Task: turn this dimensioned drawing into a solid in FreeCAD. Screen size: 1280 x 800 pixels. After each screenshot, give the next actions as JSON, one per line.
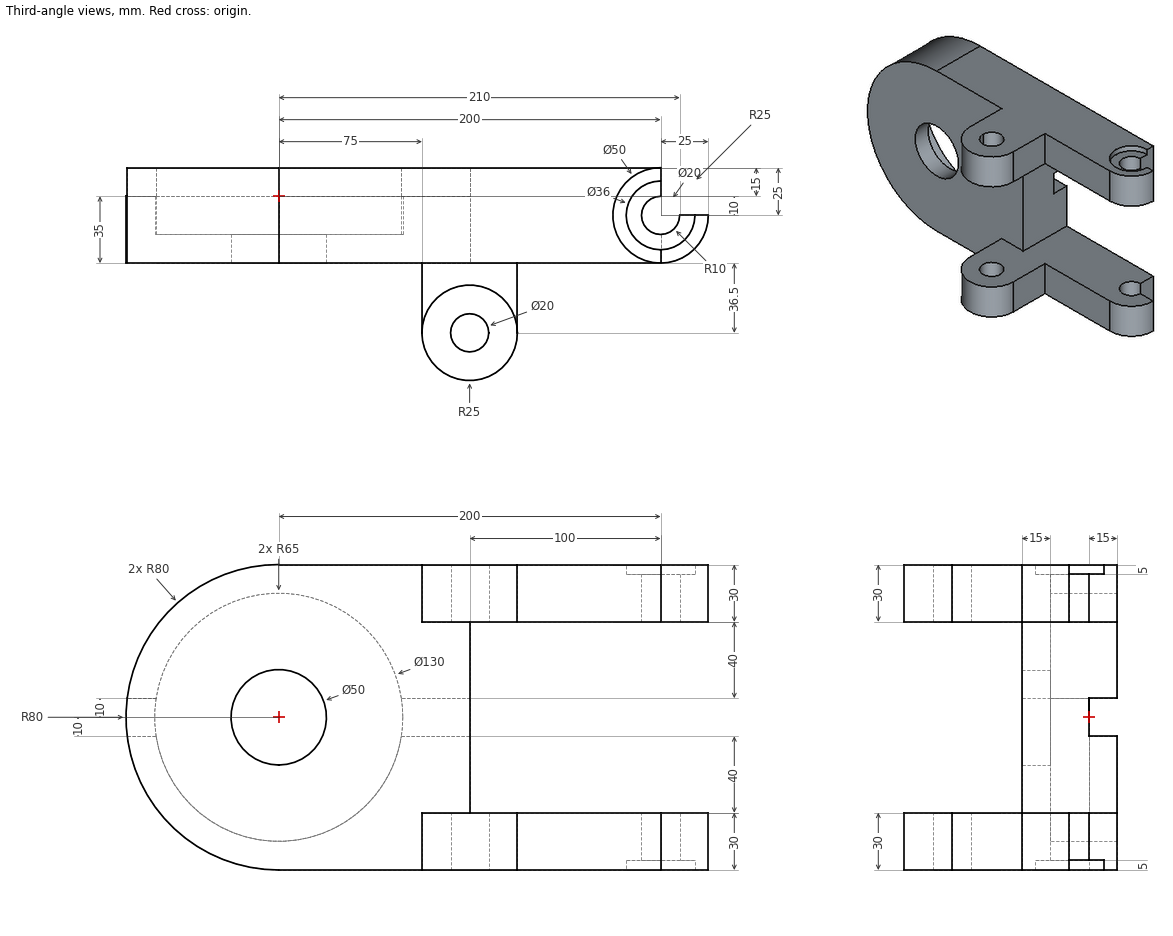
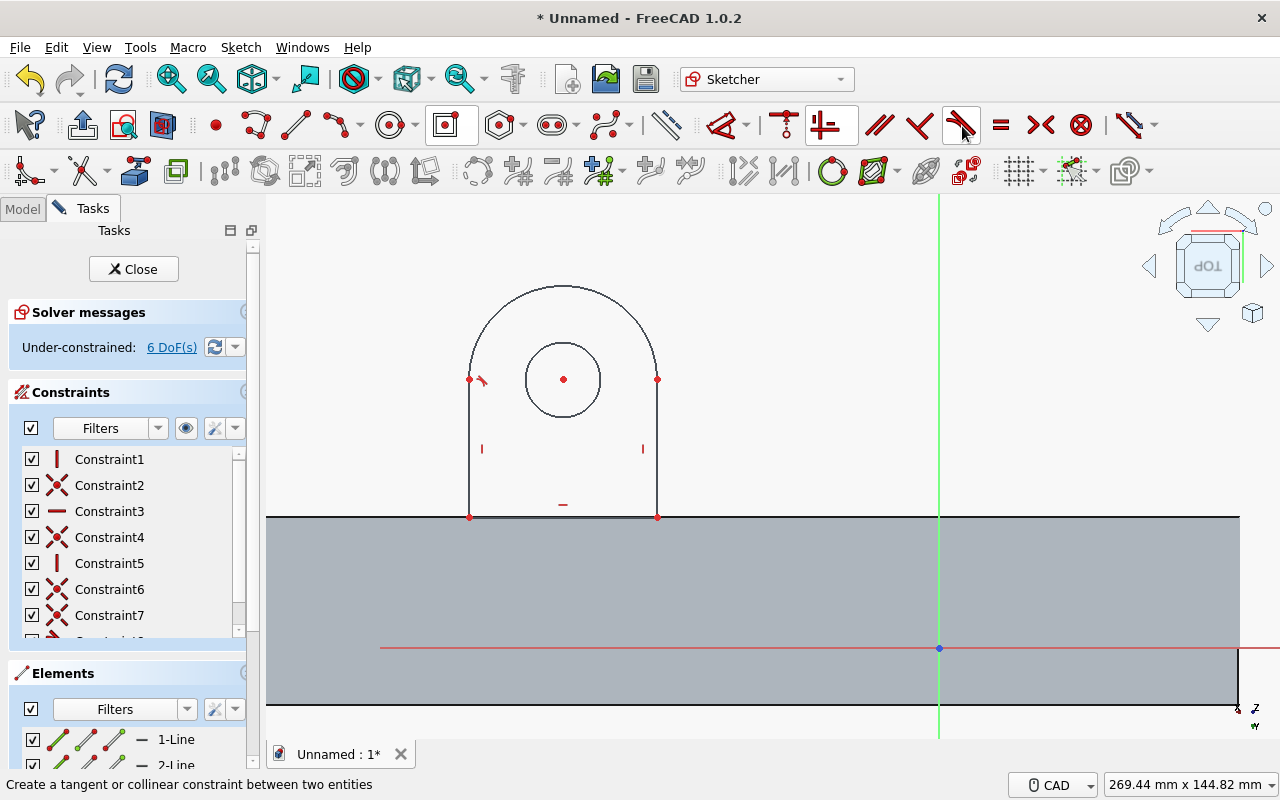
{"action": "left_click", "coordinate": [657, 477]}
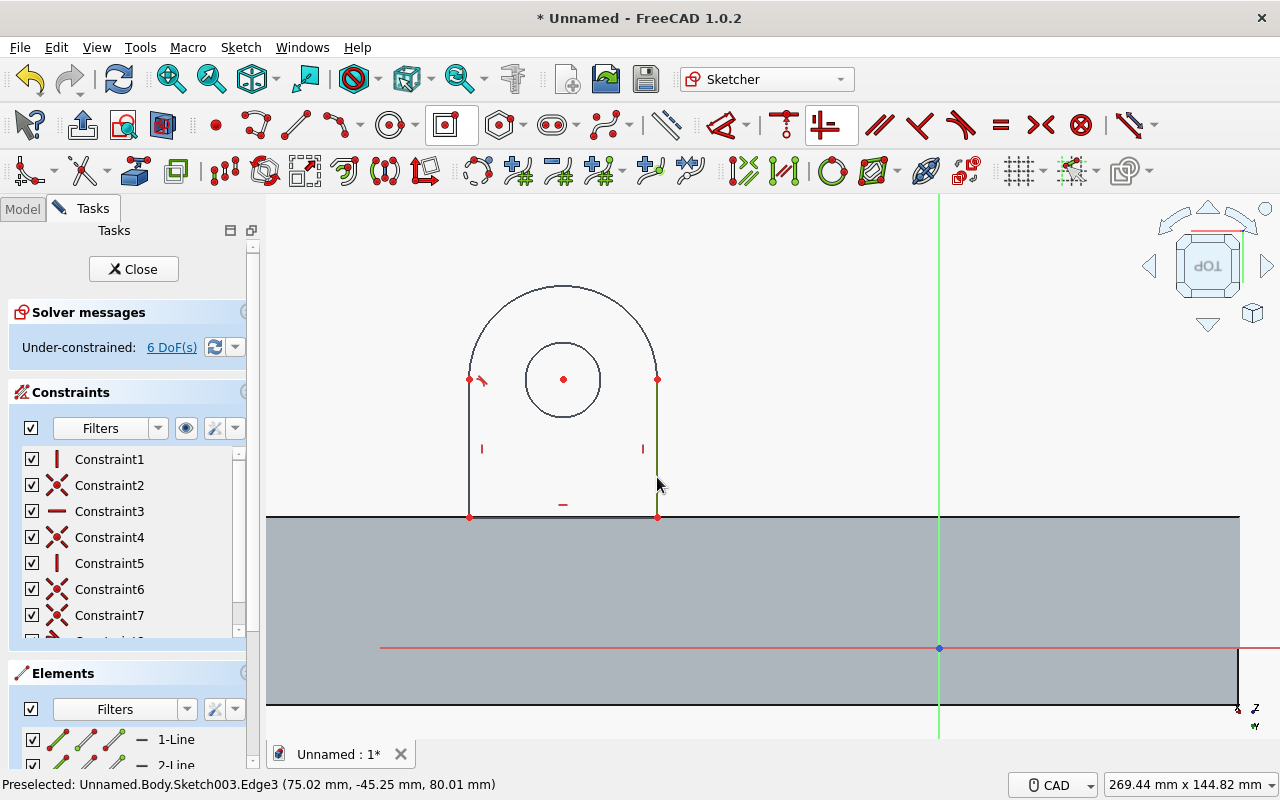
{"action": "left_click", "coordinate": [618, 304]}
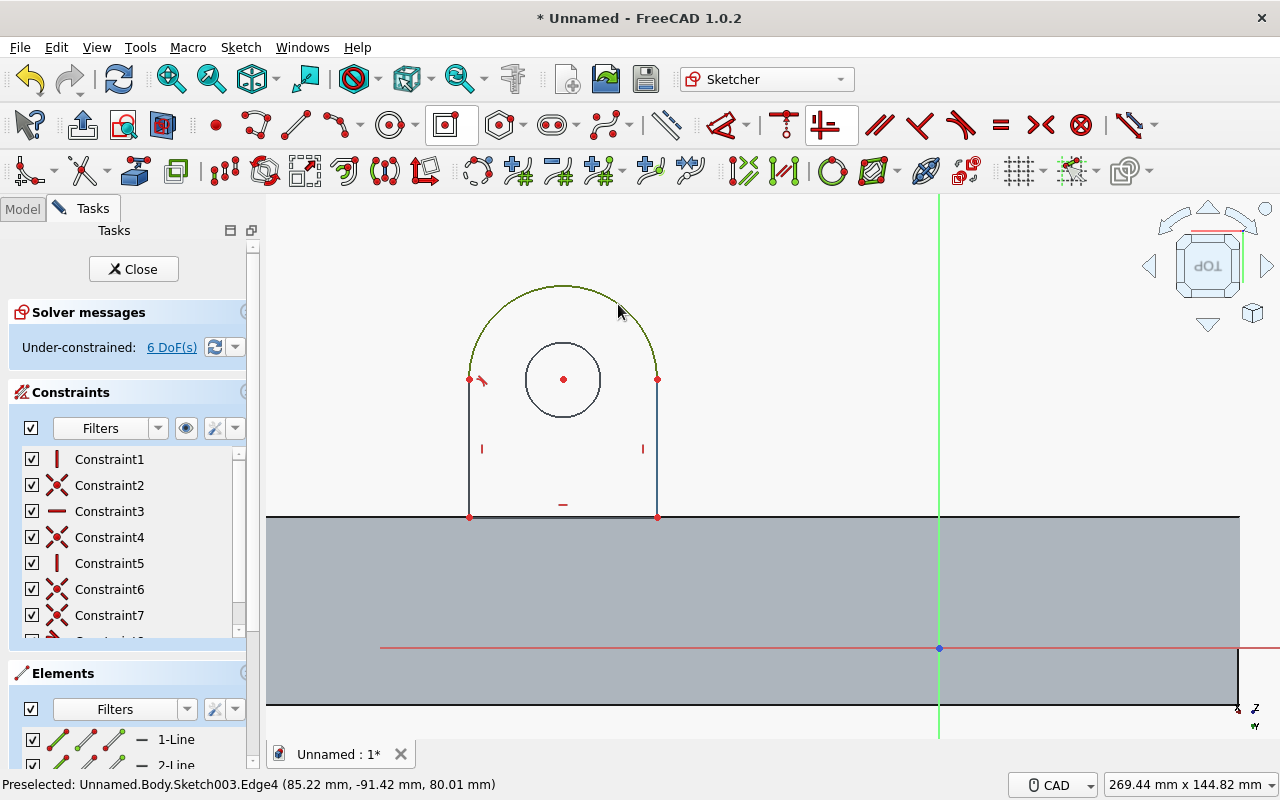
{"action": "key", "text": "t"}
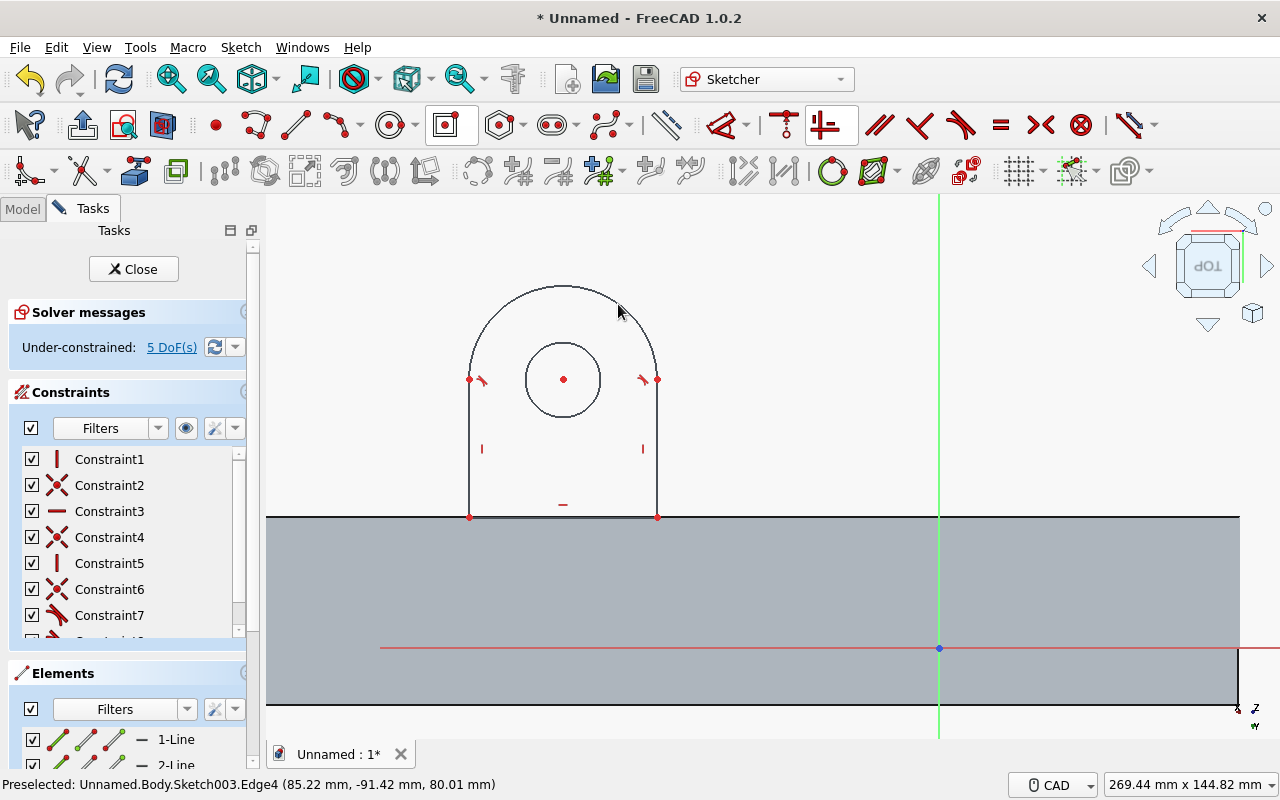
{"action": "left_click", "coordinate": [722, 126]}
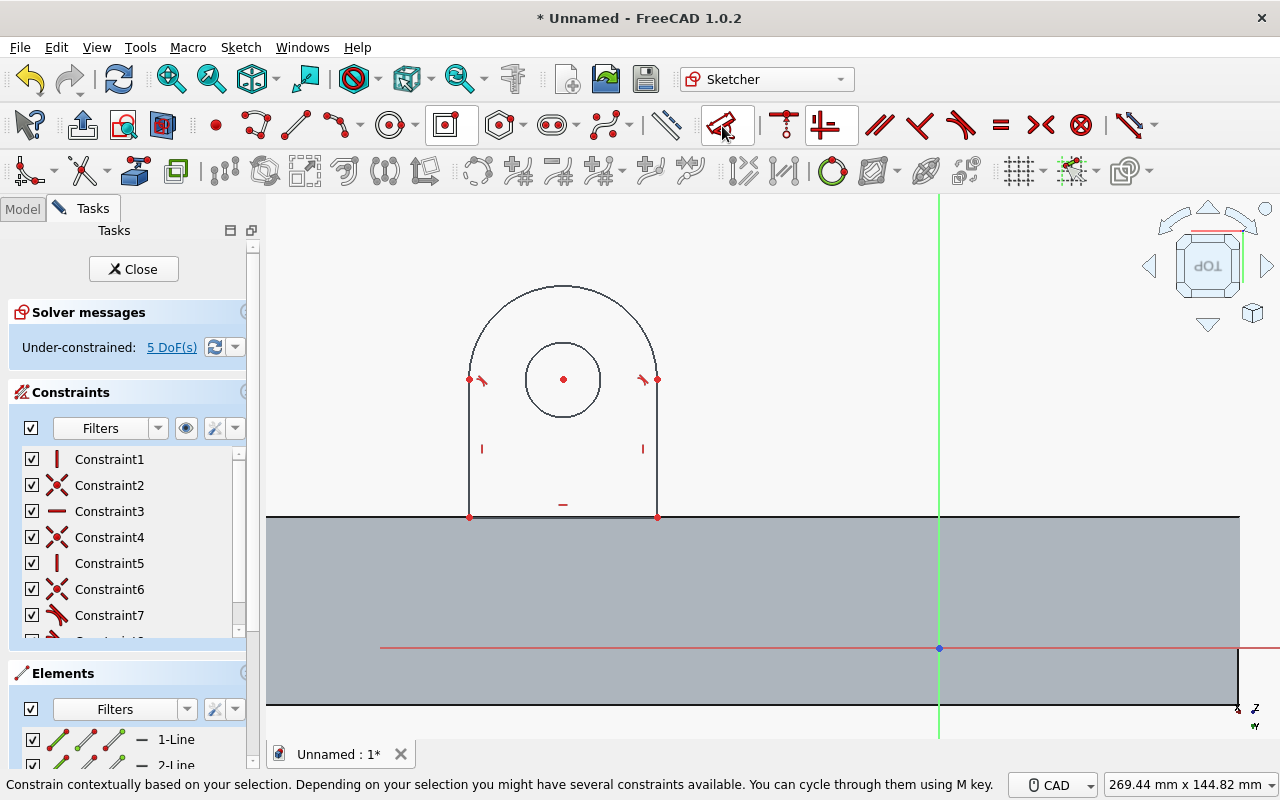
{"action": "left_click", "coordinate": [618, 304]}
{"action": "left_click", "coordinate": [637, 278]}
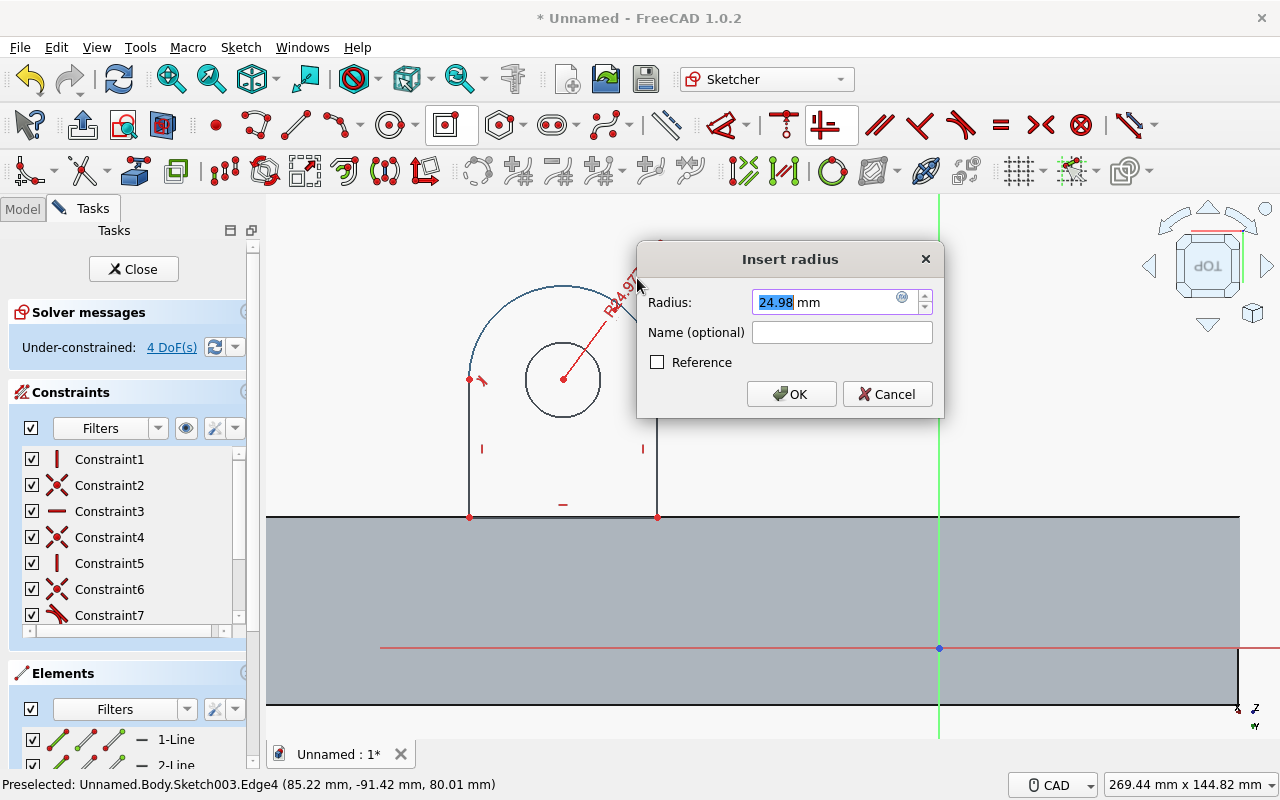
{"action": "type", "text": "25"}
{"action": "key", "text": "Return"}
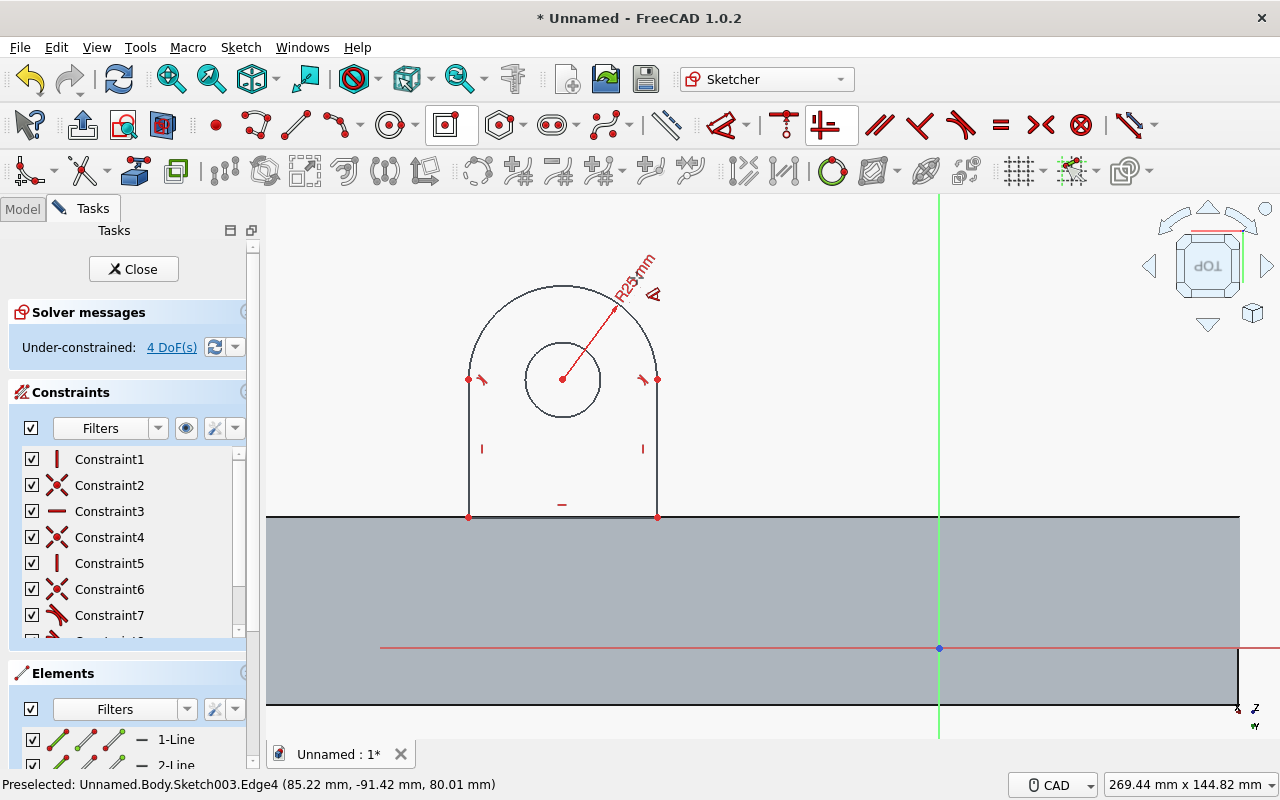
{"action": "left_click", "coordinate": [589, 353]}
{"action": "left_click", "coordinate": [611, 330]}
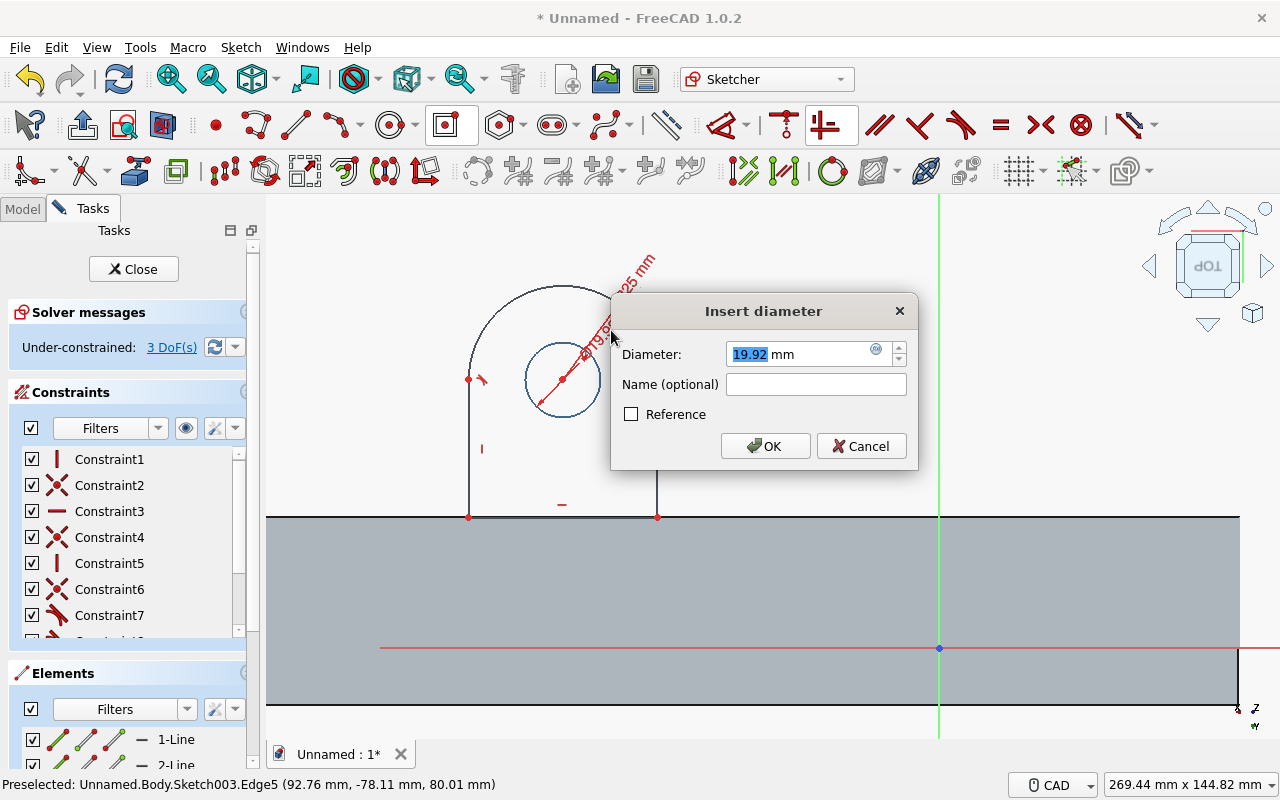
{"action": "type", "text": "20"}
{"action": "key", "text": "Return"}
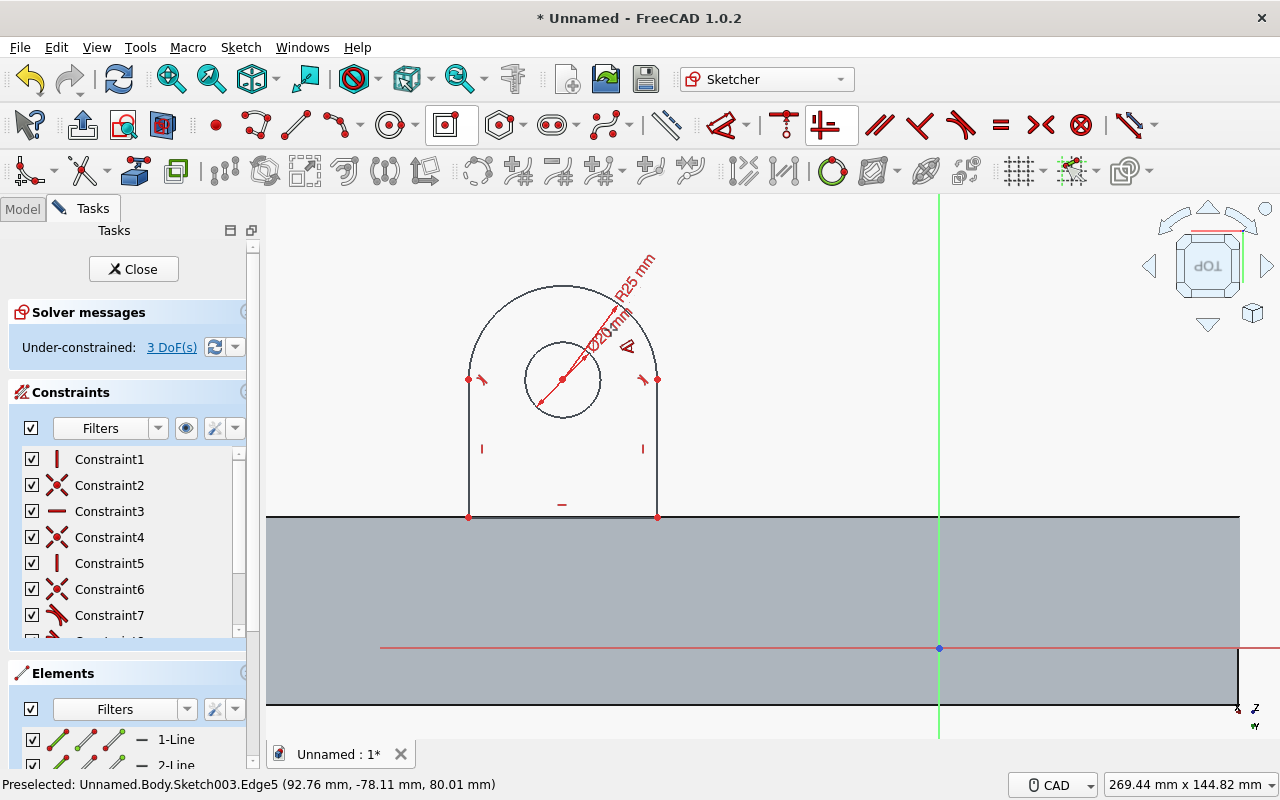
{"action": "left_click", "coordinate": [469, 518]}
{"action": "left_click", "coordinate": [435, 583]}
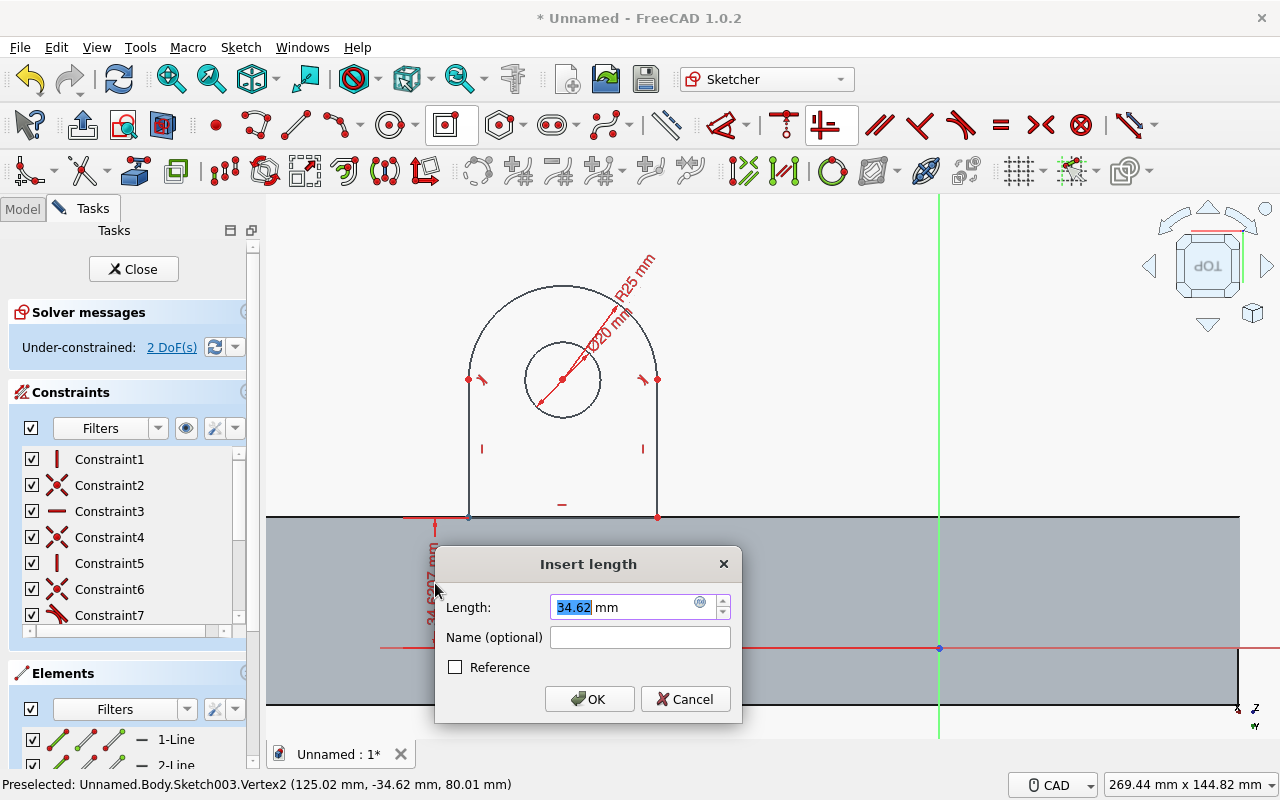
{"action": "type", "text": "35"}
{"action": "key", "text": "Return"}